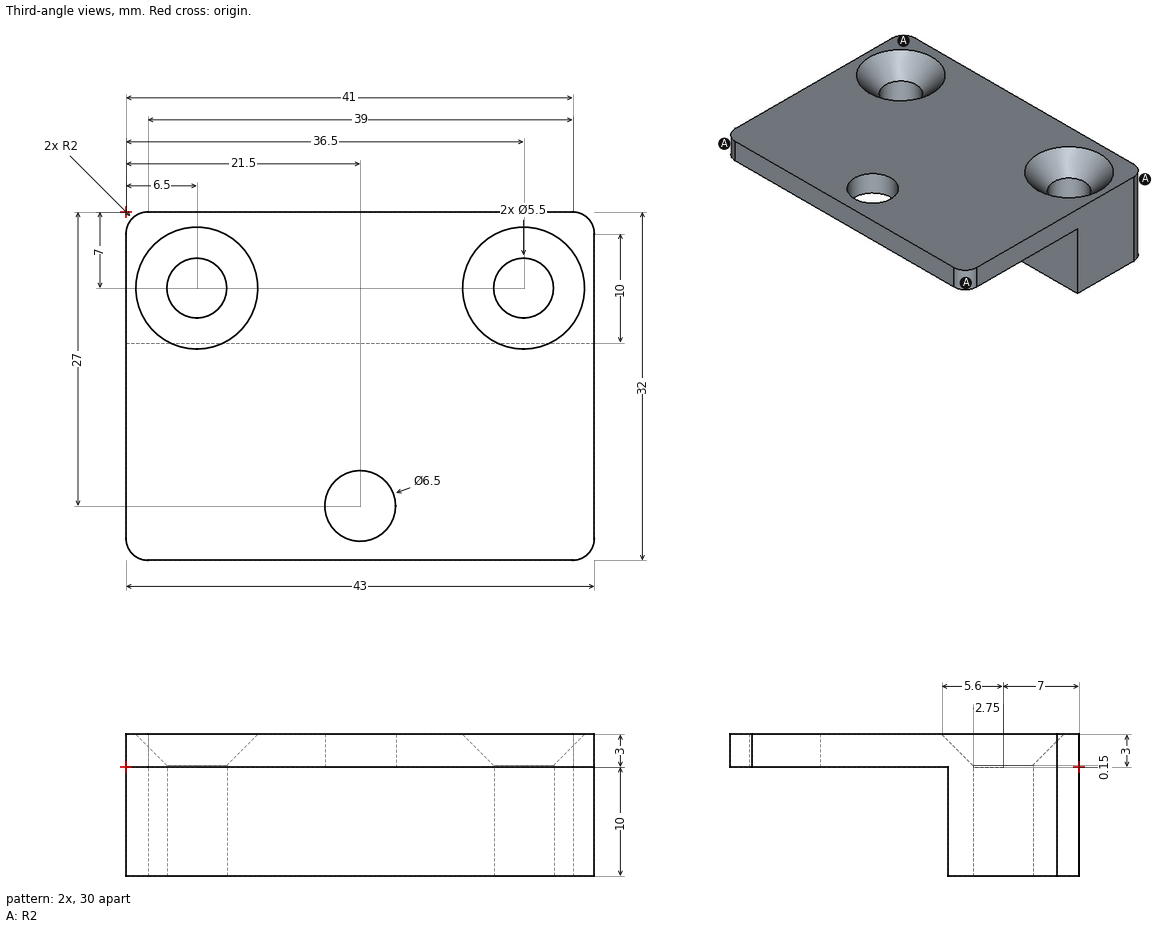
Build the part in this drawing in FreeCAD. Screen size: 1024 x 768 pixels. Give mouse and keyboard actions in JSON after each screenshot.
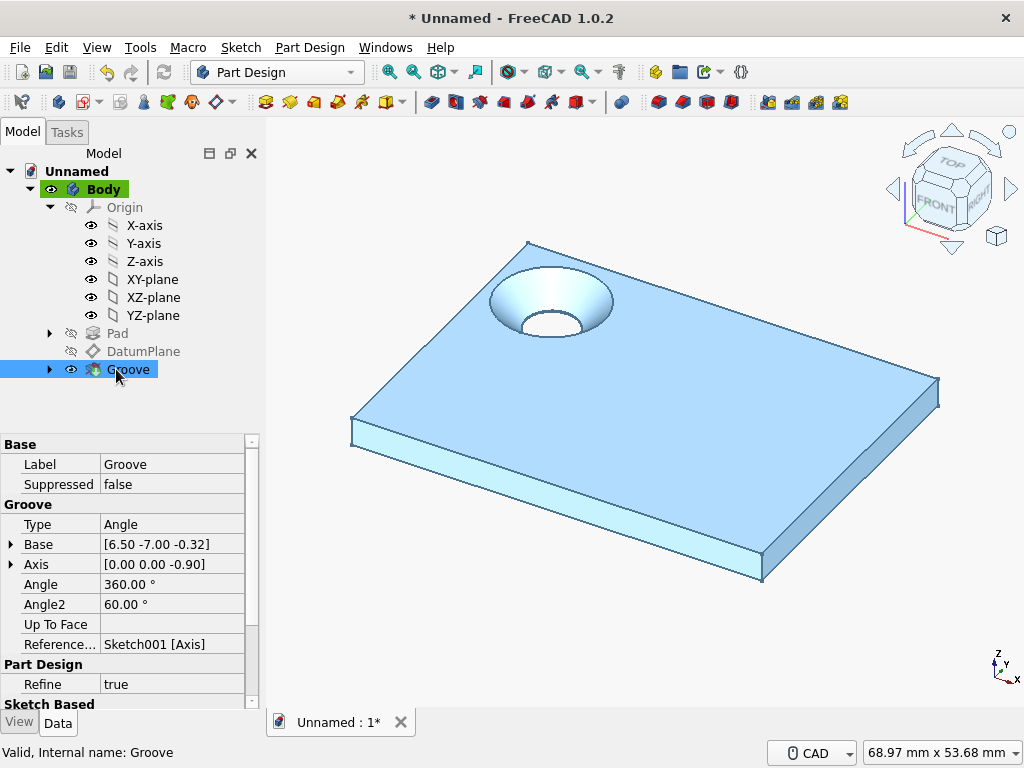
{"action": "left_click", "coordinate": [792, 102]}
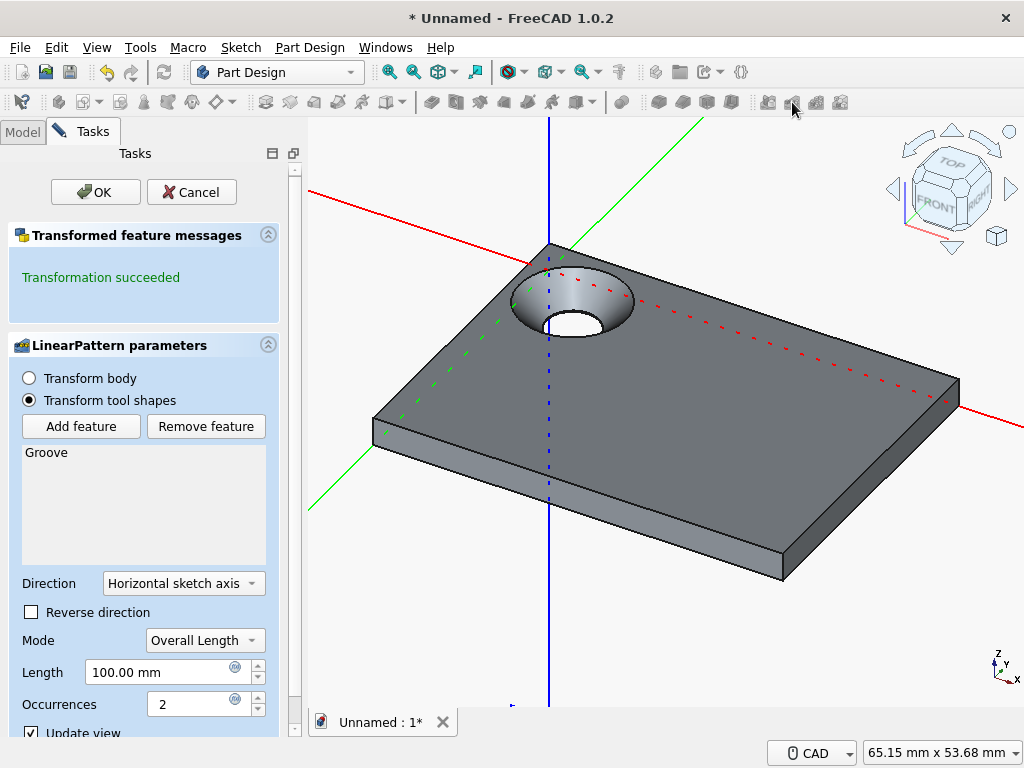
{"action": "left_click", "coordinate": [184, 584]}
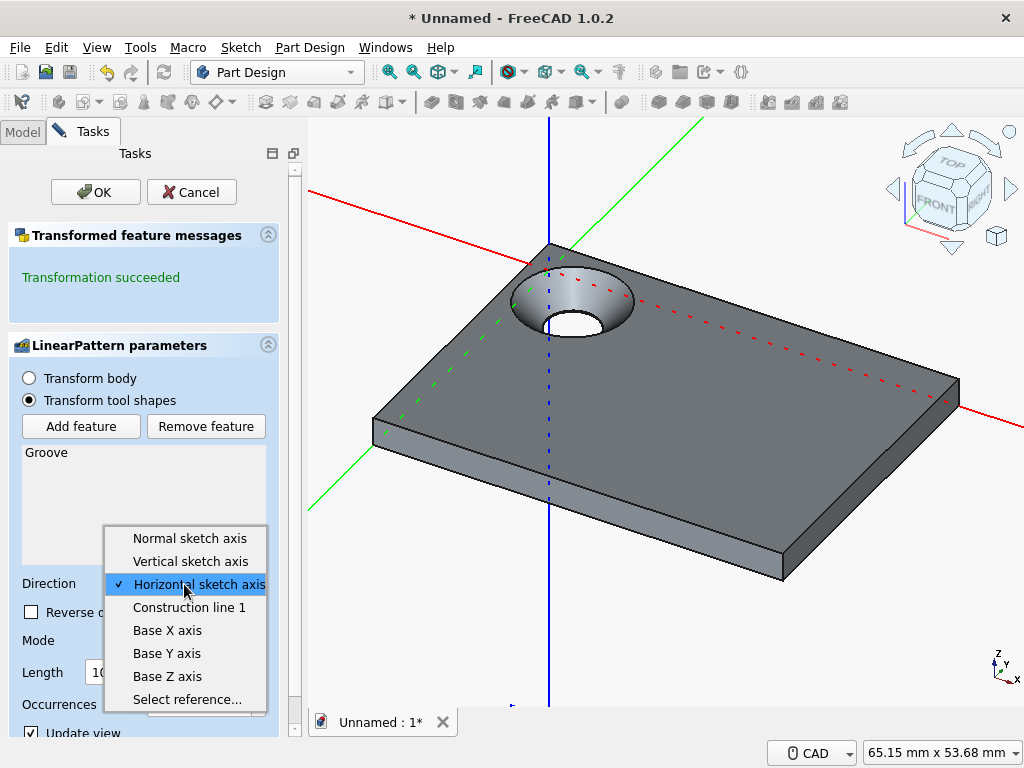
{"action": "left_click", "coordinate": [184, 630]}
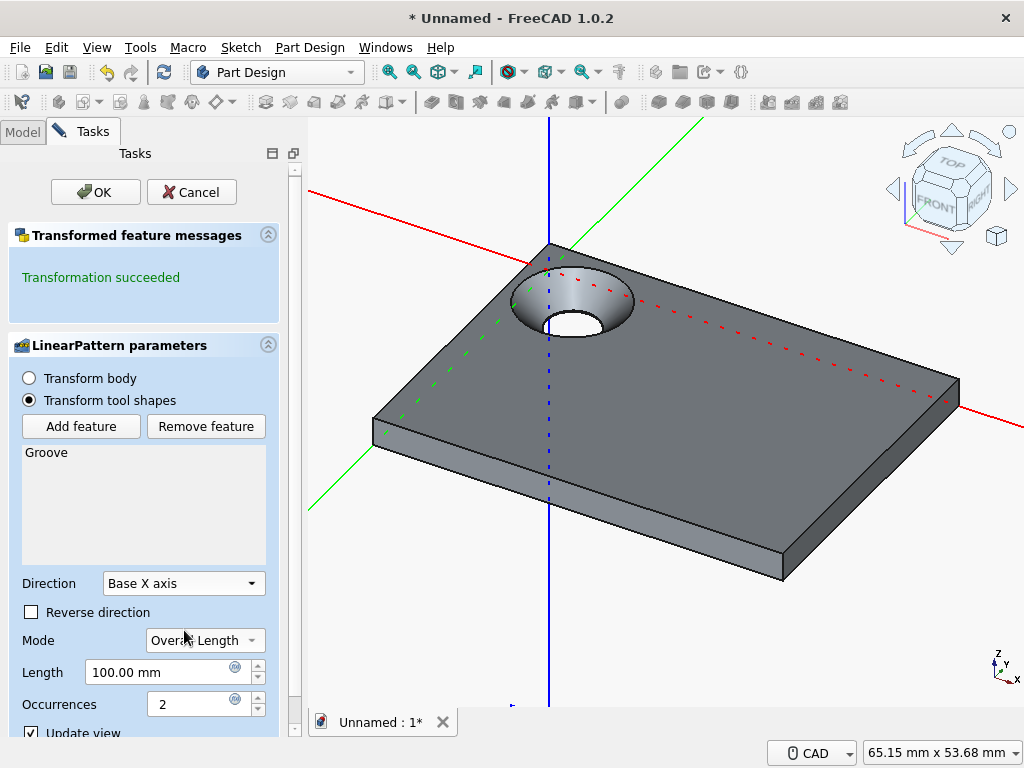
{"action": "left_click", "coordinate": [206, 640]}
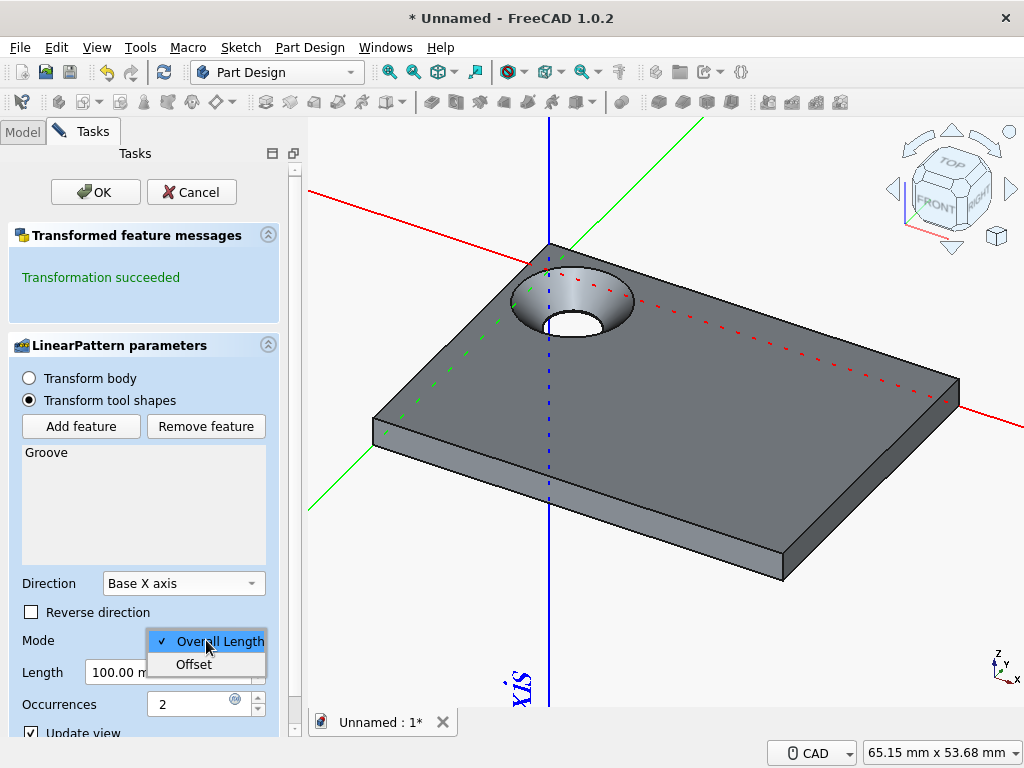
{"action": "left_click", "coordinate": [206, 664]}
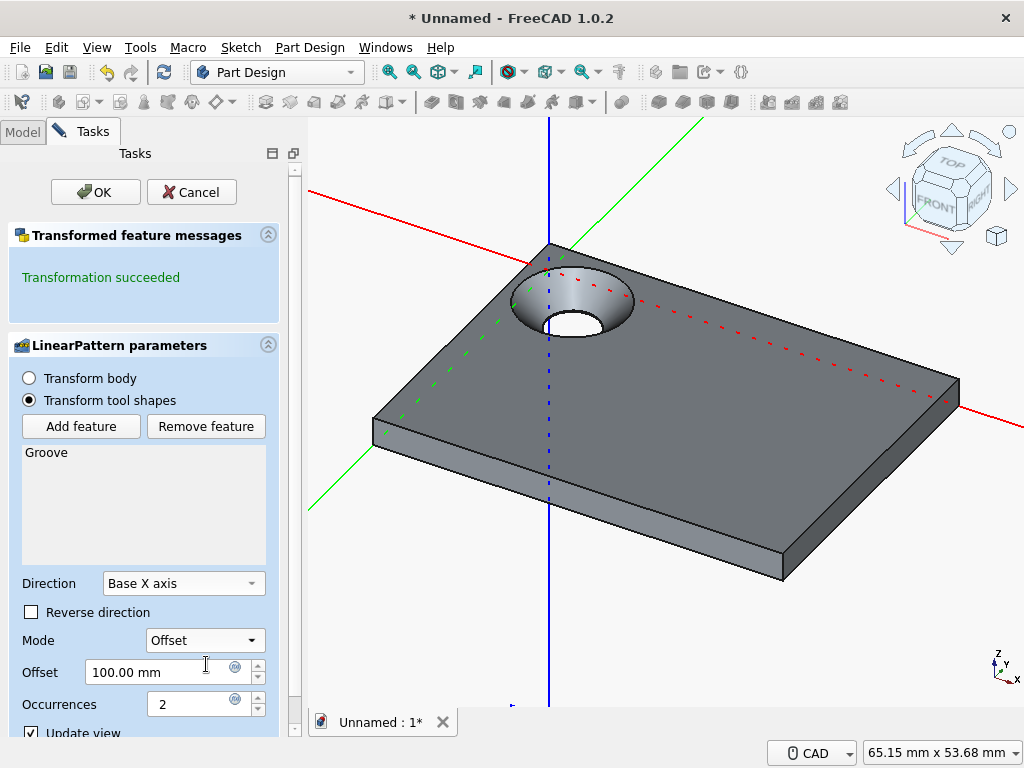
{"action": "triple_click", "coordinate": [168, 672]}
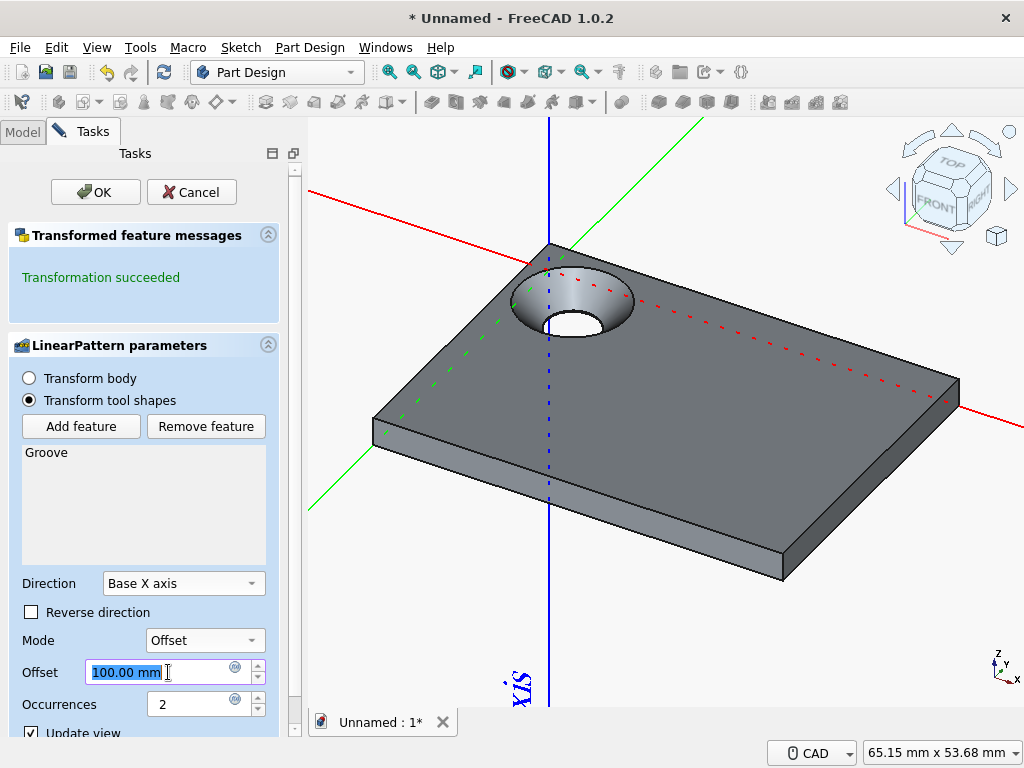
{"action": "type", "text": "30"}
{"action": "key", "text": "Tab"}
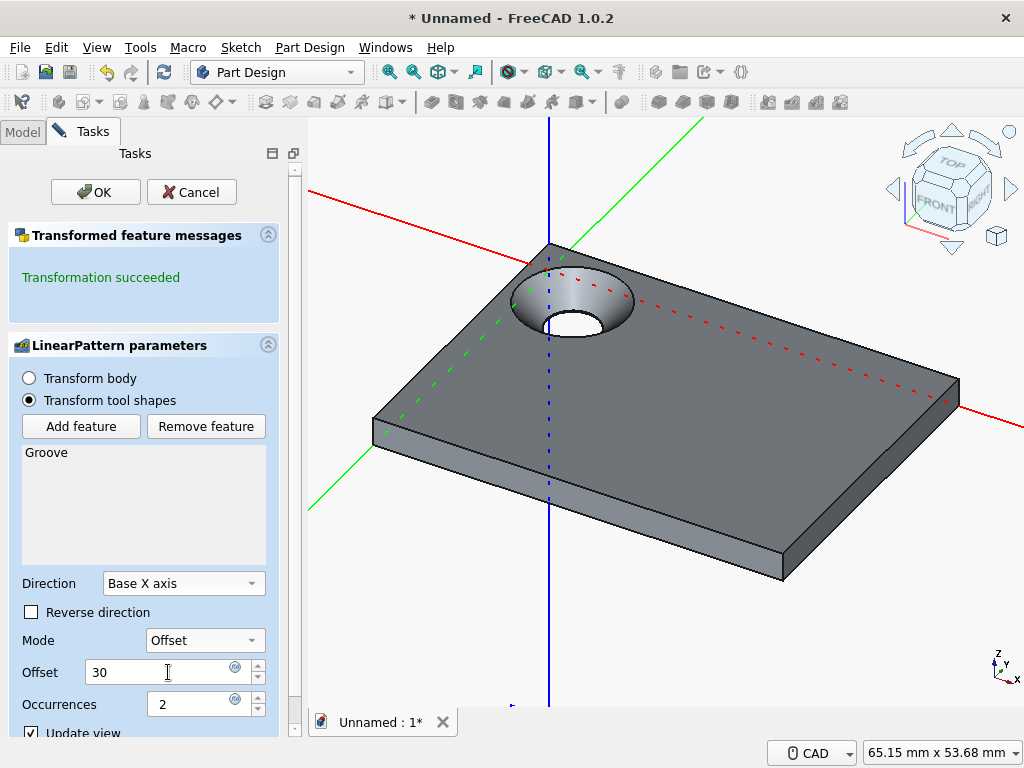
{"action": "triple_click", "coordinate": [198, 704]}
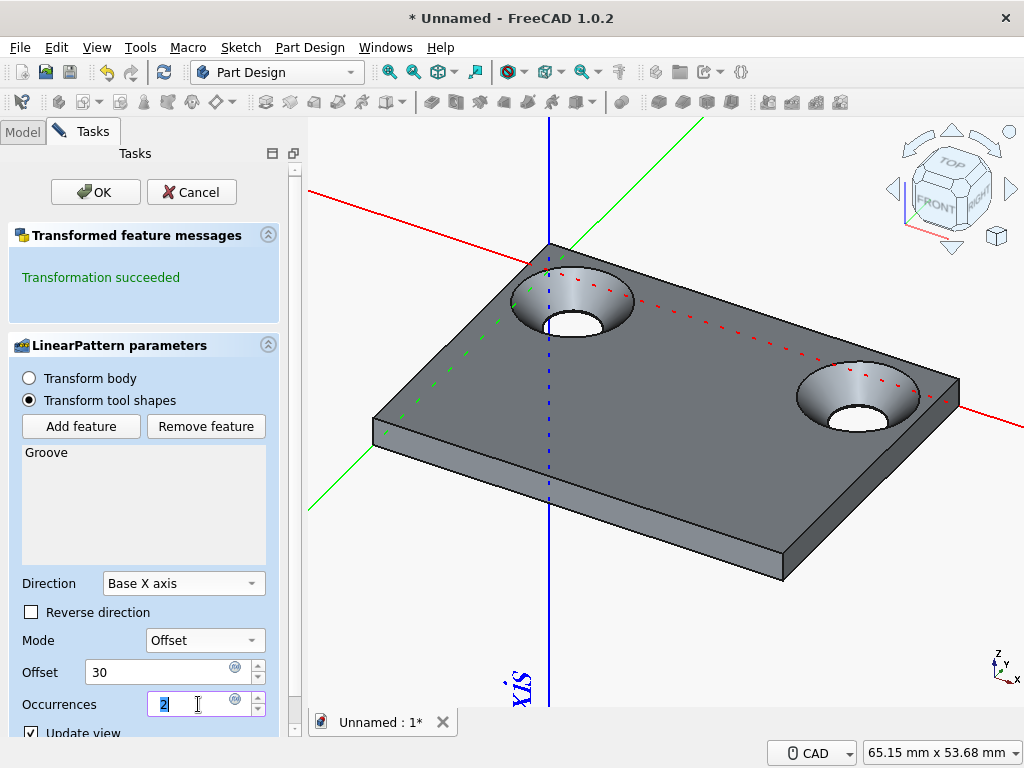
{"action": "type", "text": "2"}
{"action": "key", "text": "Tab"}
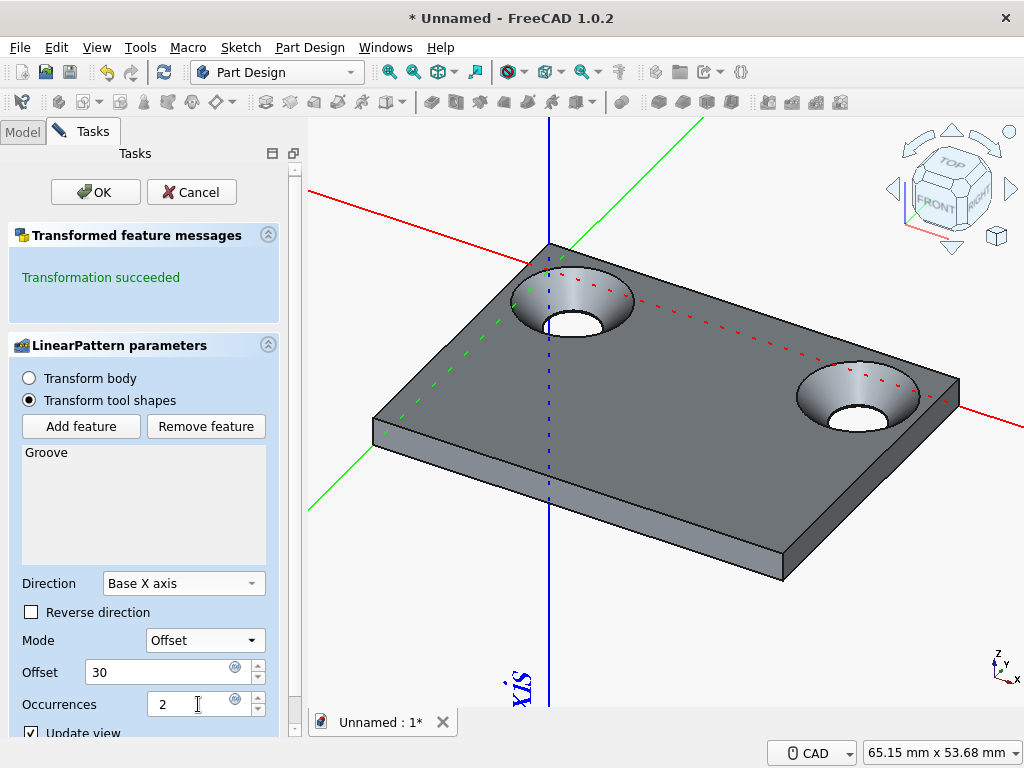
{"action": "left_click", "coordinate": [96, 192]}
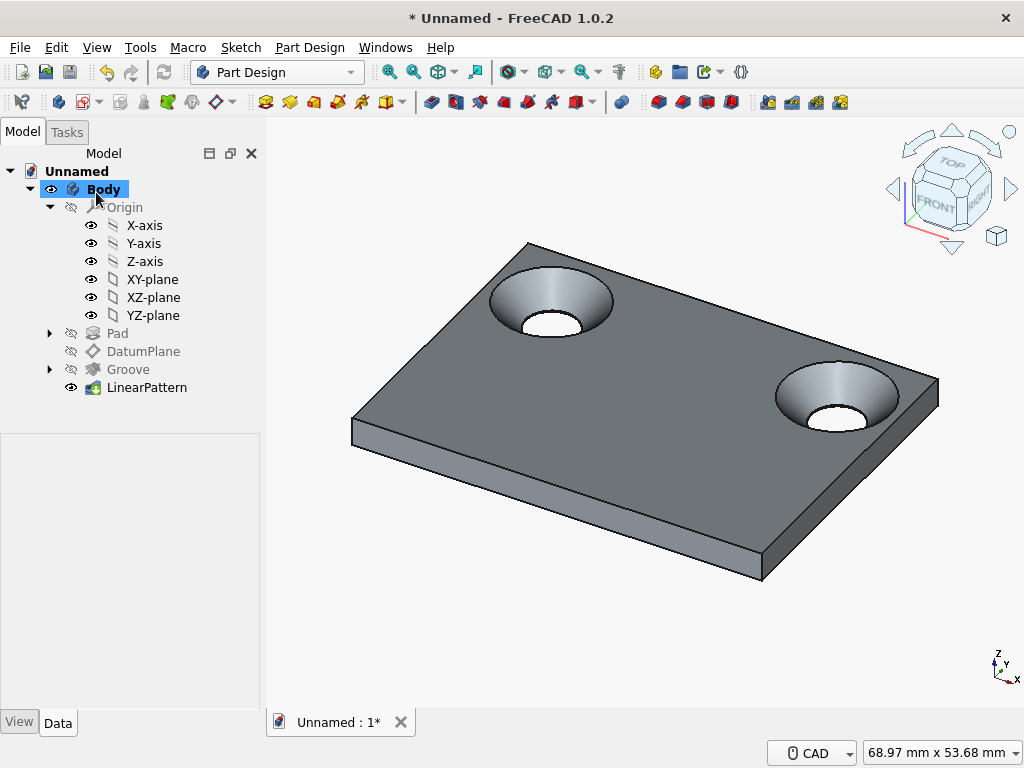
{"action": "left_click", "coordinate": [645, 397]}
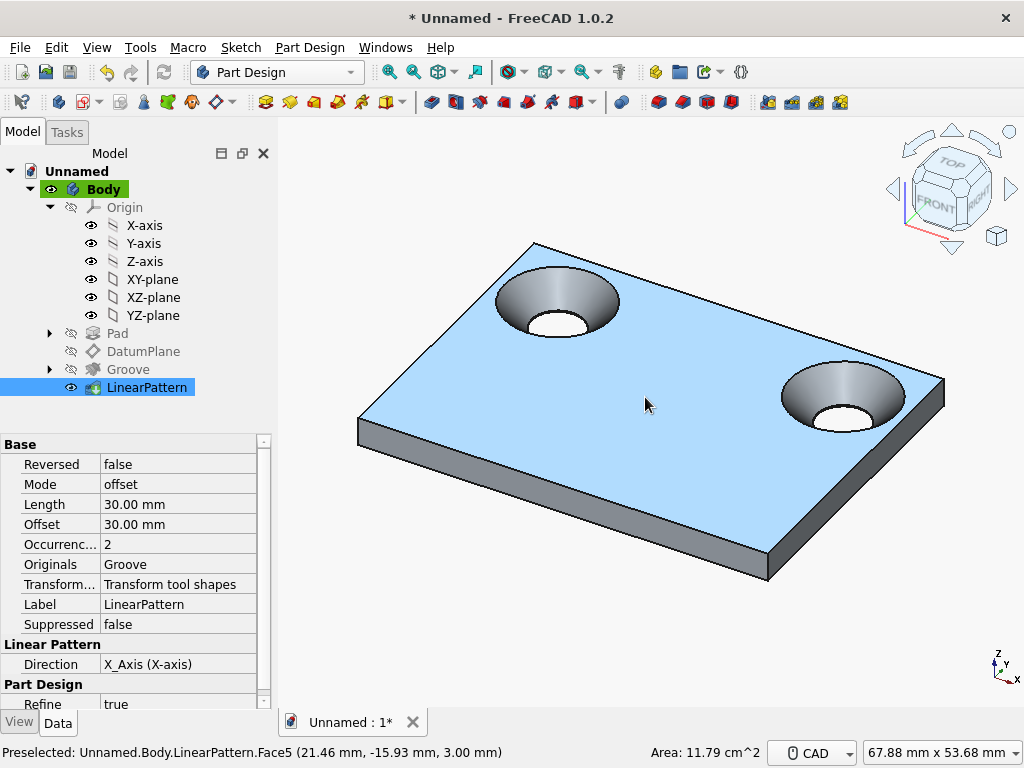
{"action": "left_click", "coordinate": [84, 102]}